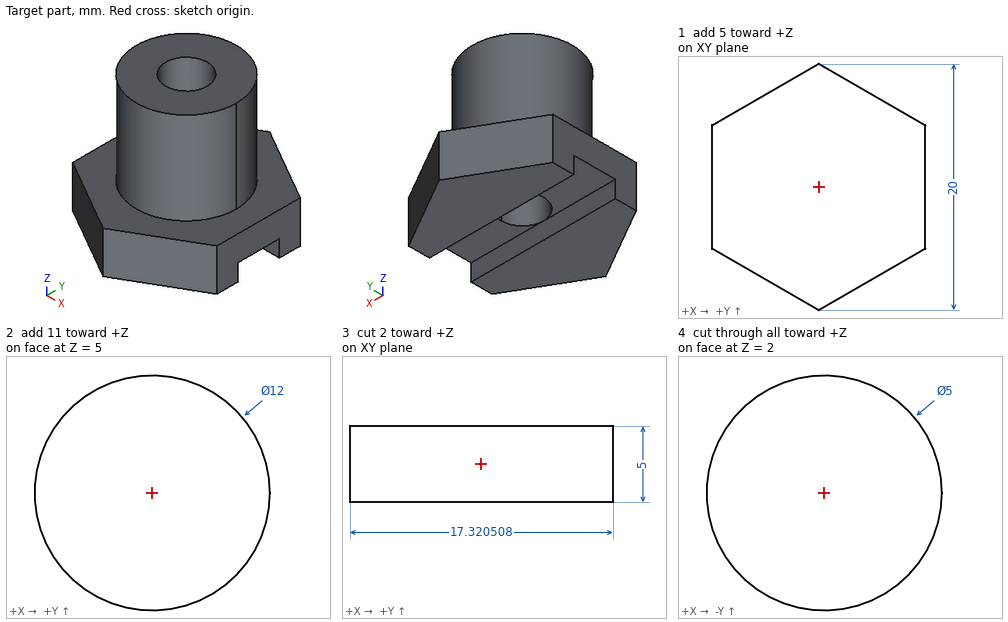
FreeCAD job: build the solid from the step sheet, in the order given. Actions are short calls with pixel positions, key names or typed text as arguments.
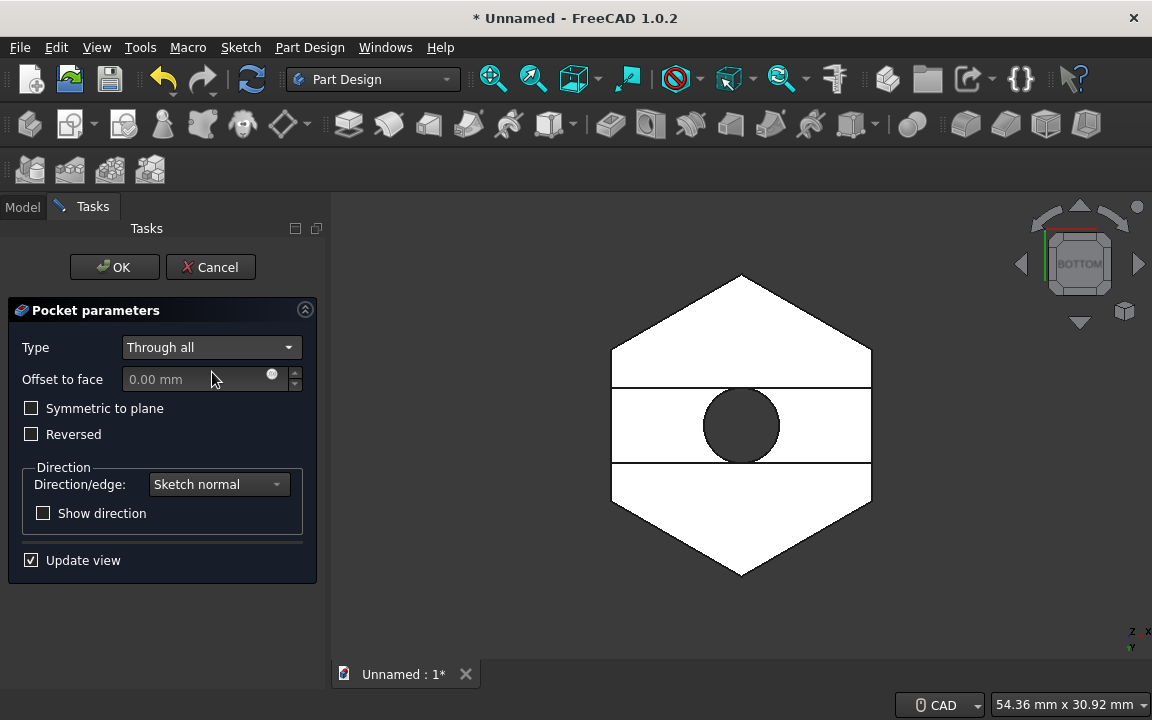
click(115, 267)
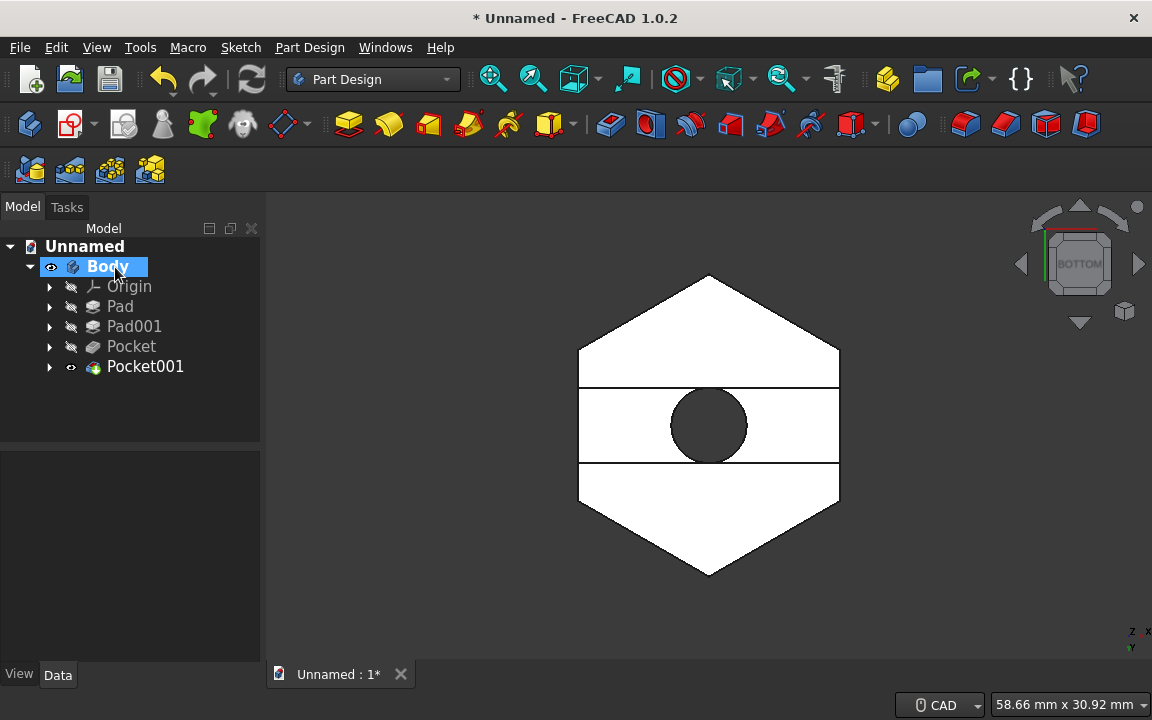
key(0)